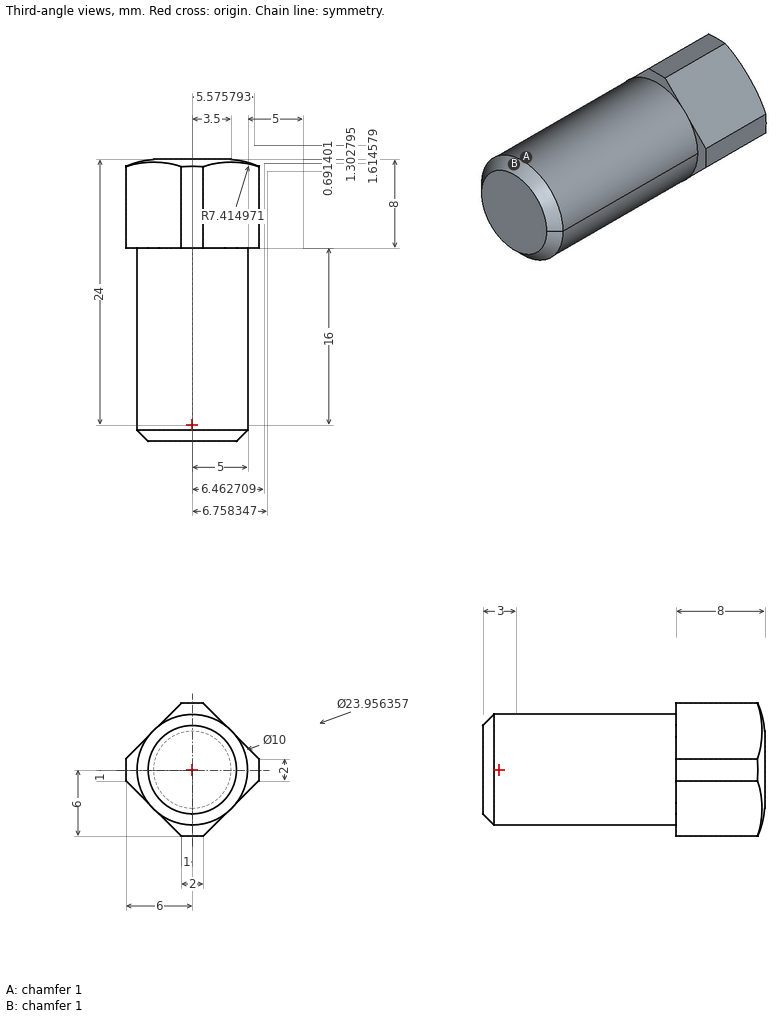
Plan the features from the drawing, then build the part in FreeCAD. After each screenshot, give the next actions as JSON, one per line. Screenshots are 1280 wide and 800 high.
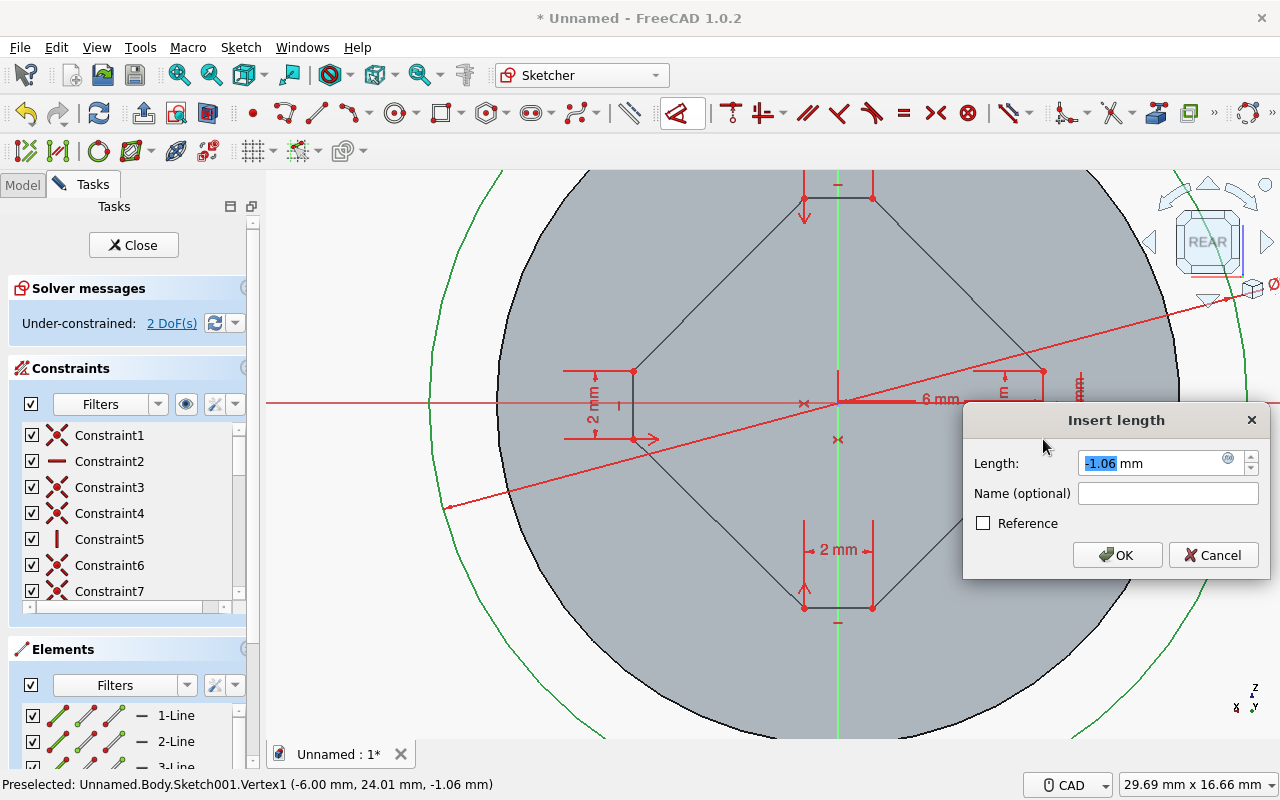
{"action": "type", "text": "-1"}
{"action": "key", "text": "Return"}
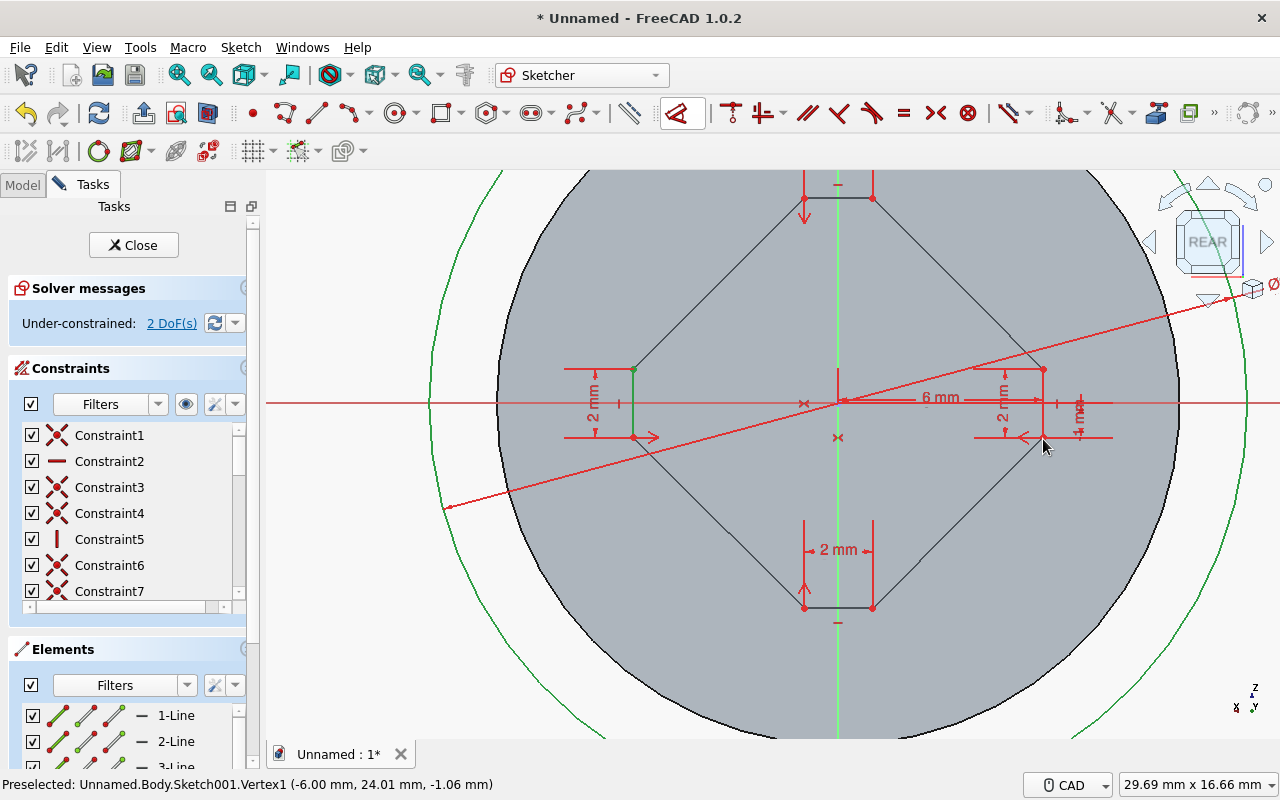
{"action": "left_click", "coordinate": [873, 608]}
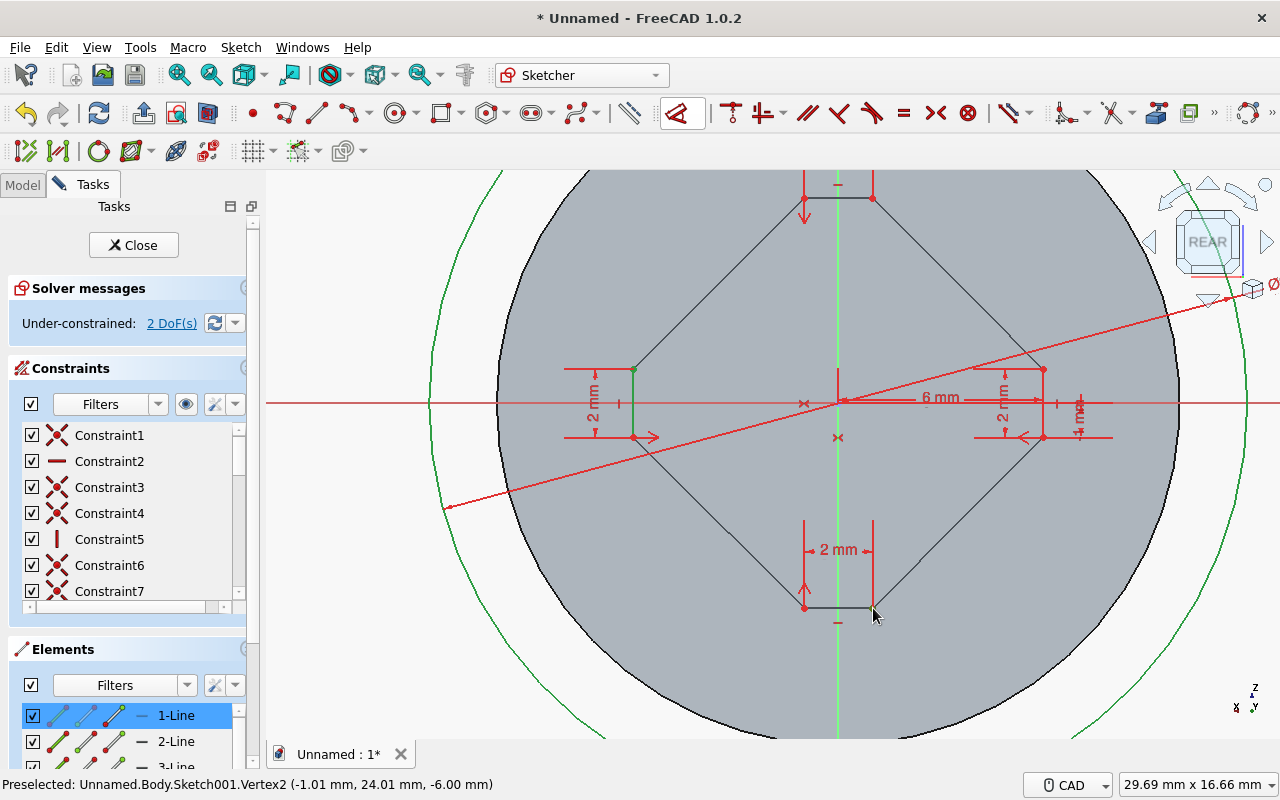
{"action": "key", "text": "l"}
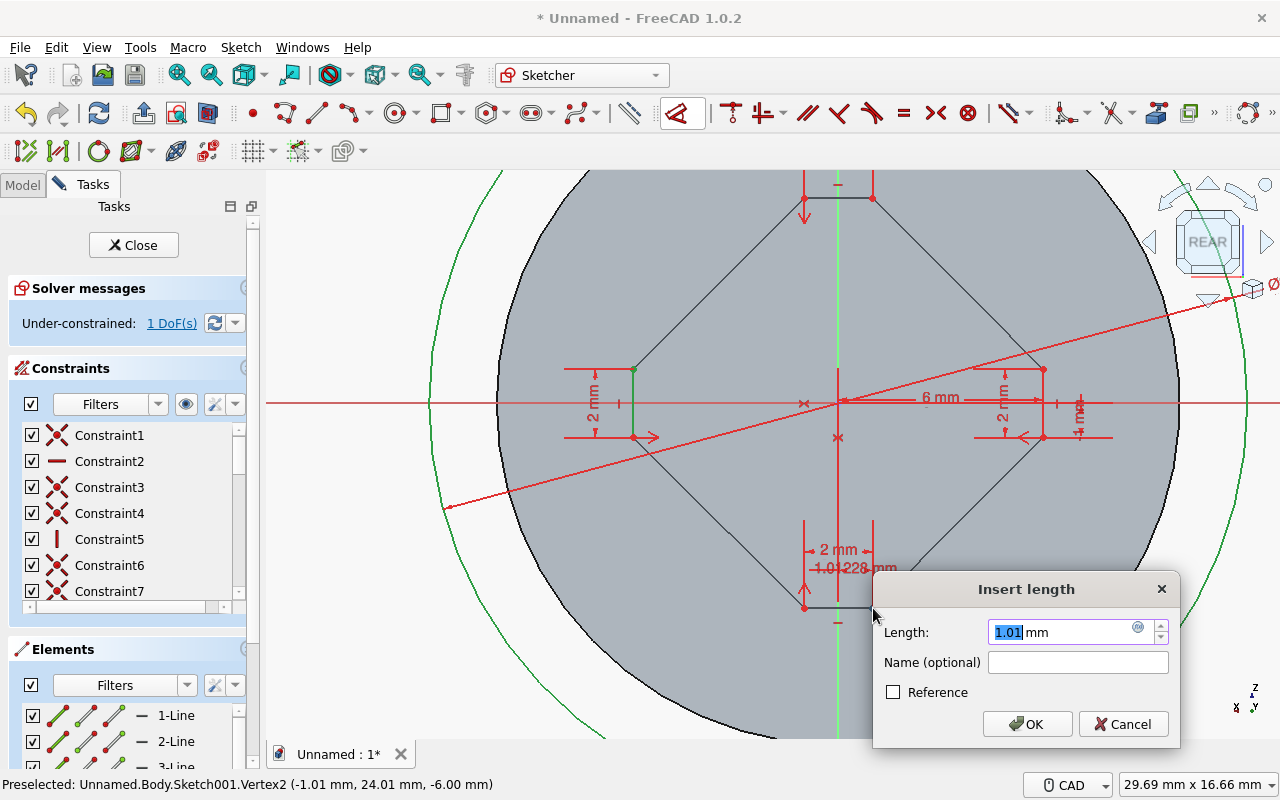
{"action": "type", "text": "1"}
{"action": "key", "text": "Return"}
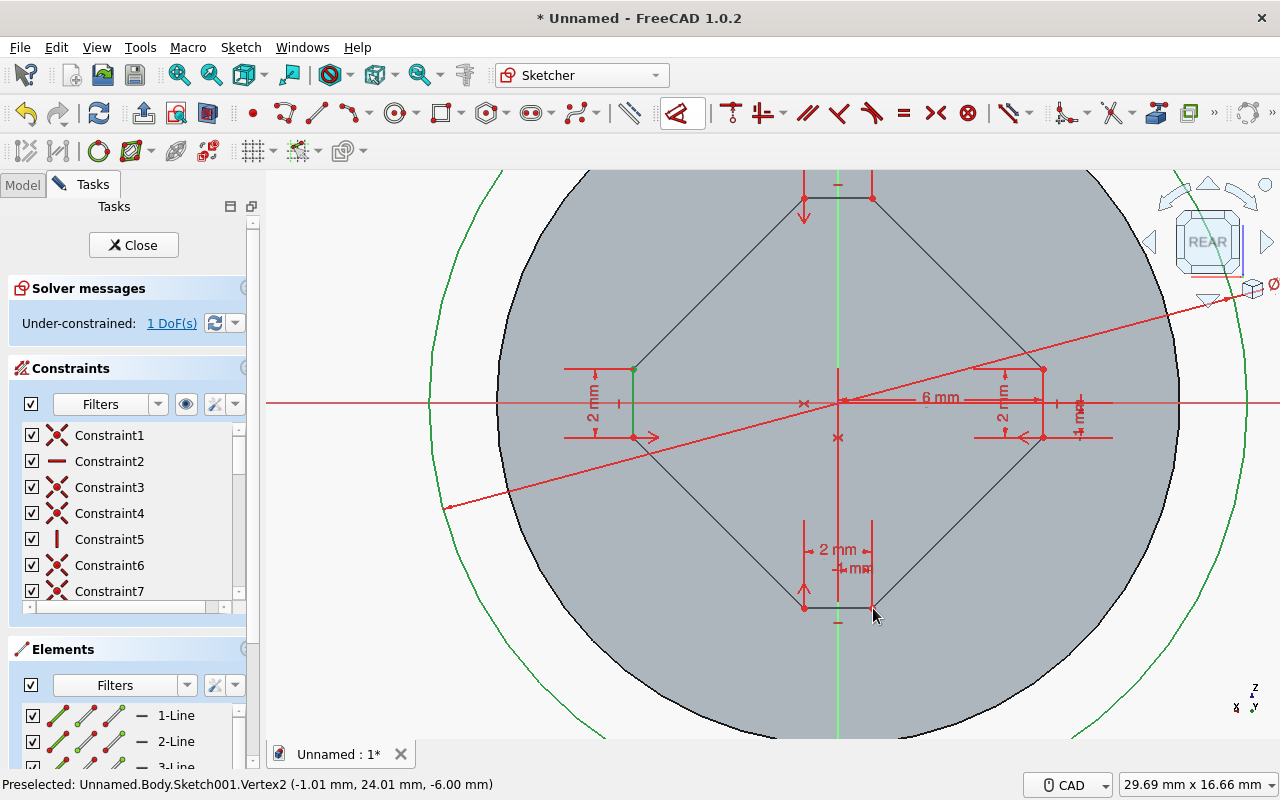
{"action": "left_click", "coordinate": [872, 608]}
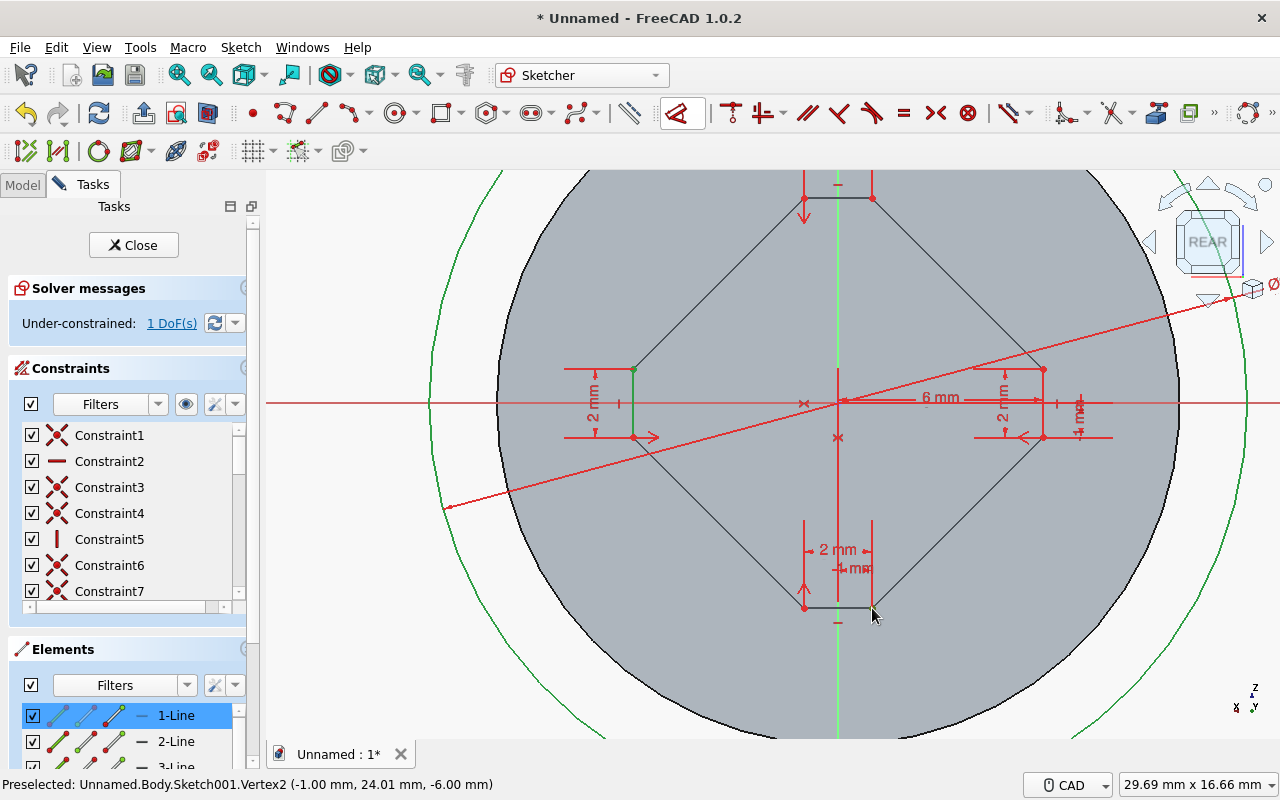
{"action": "key", "text": "i"}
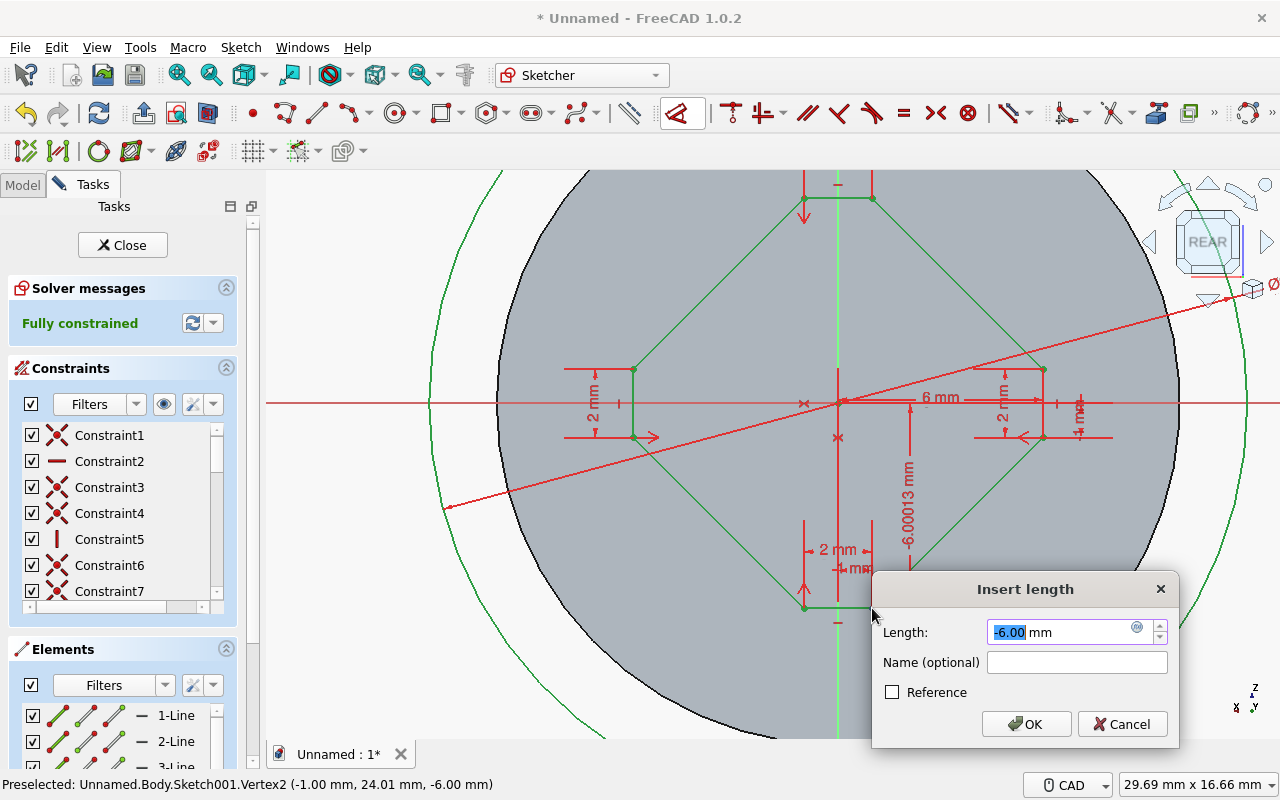
{"action": "type", "text": "-6"}
{"action": "key", "text": "Return"}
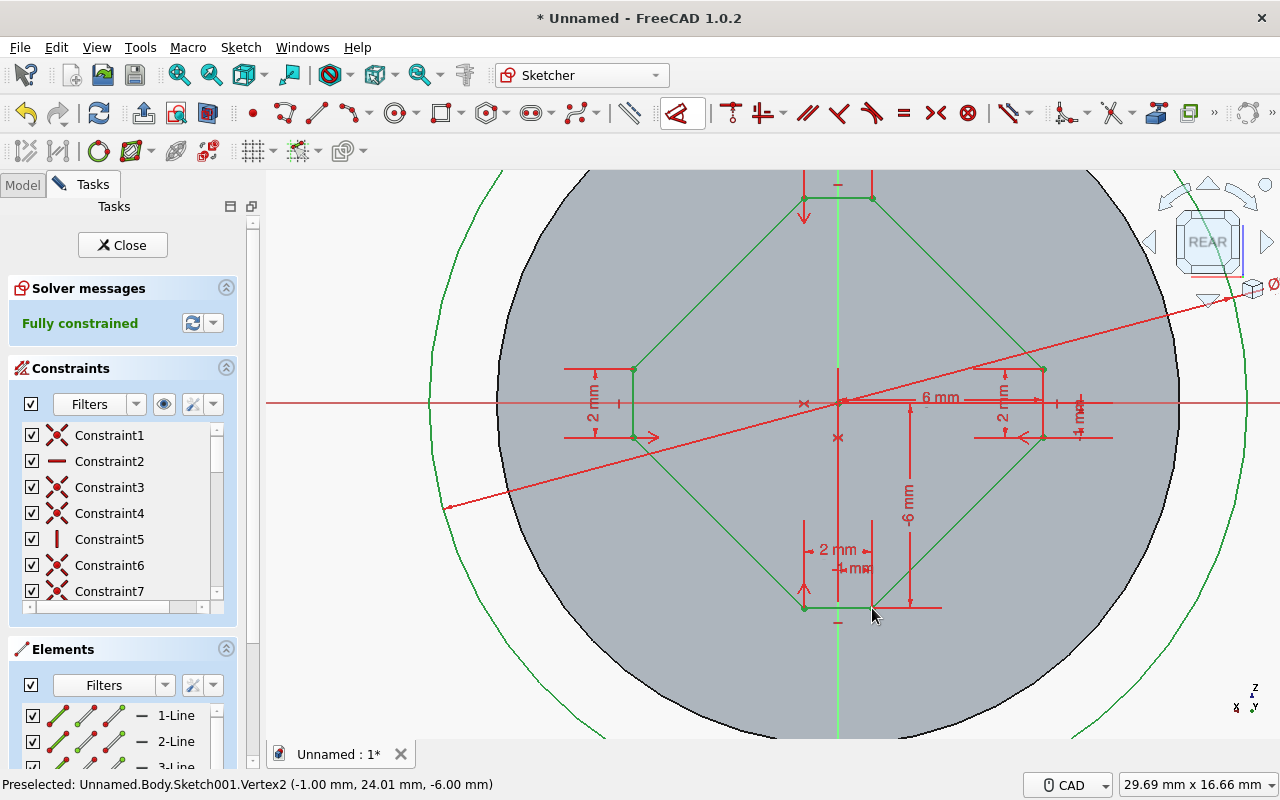
{"action": "left_click", "coordinate": [123, 245]}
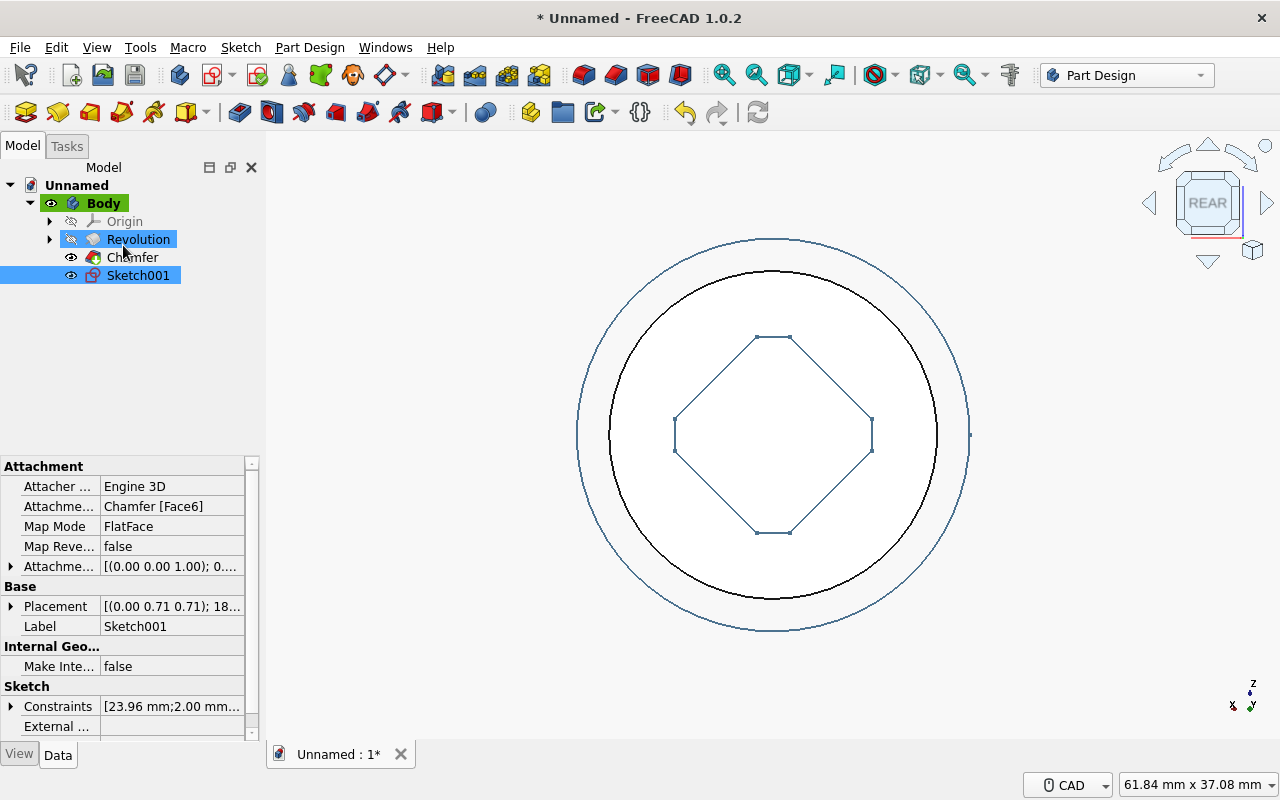
{"action": "left_click", "coordinate": [240, 112]}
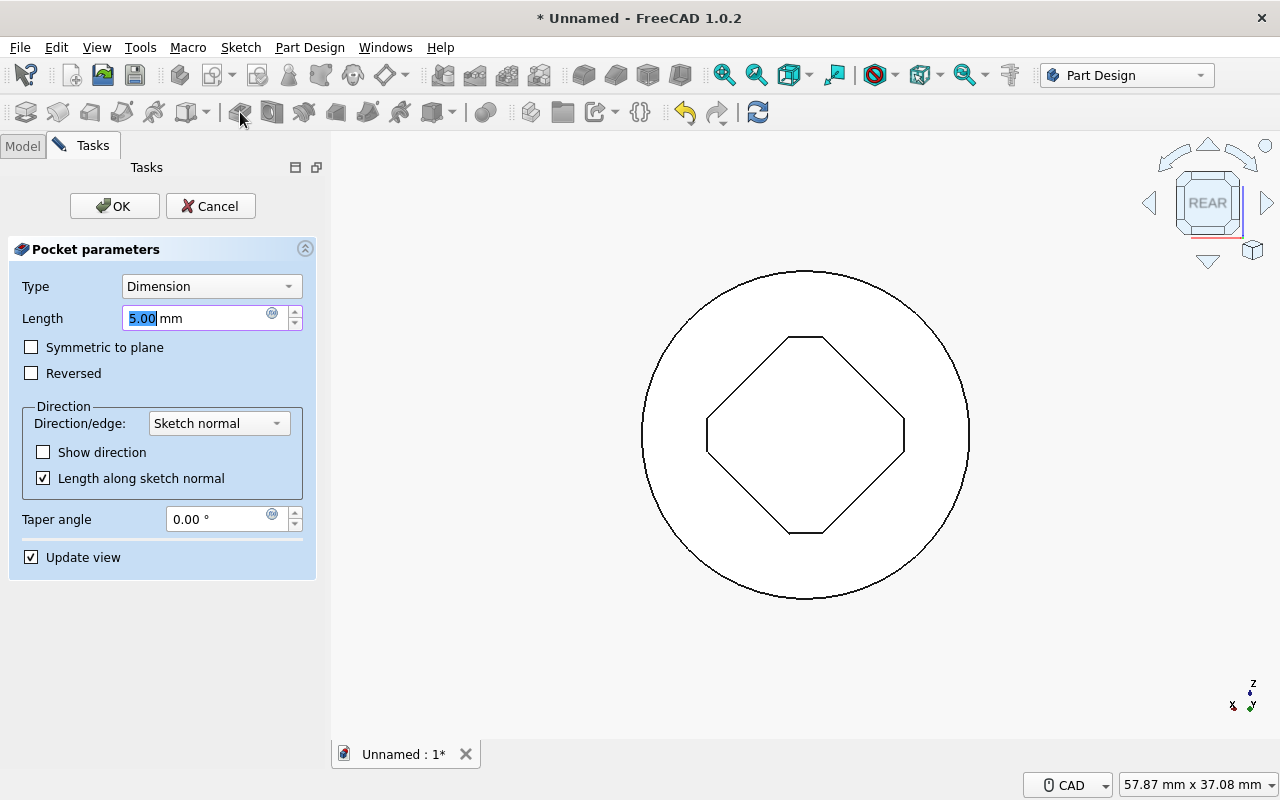
{"action": "type", "text": "8"}
{"action": "key", "text": "Tab"}